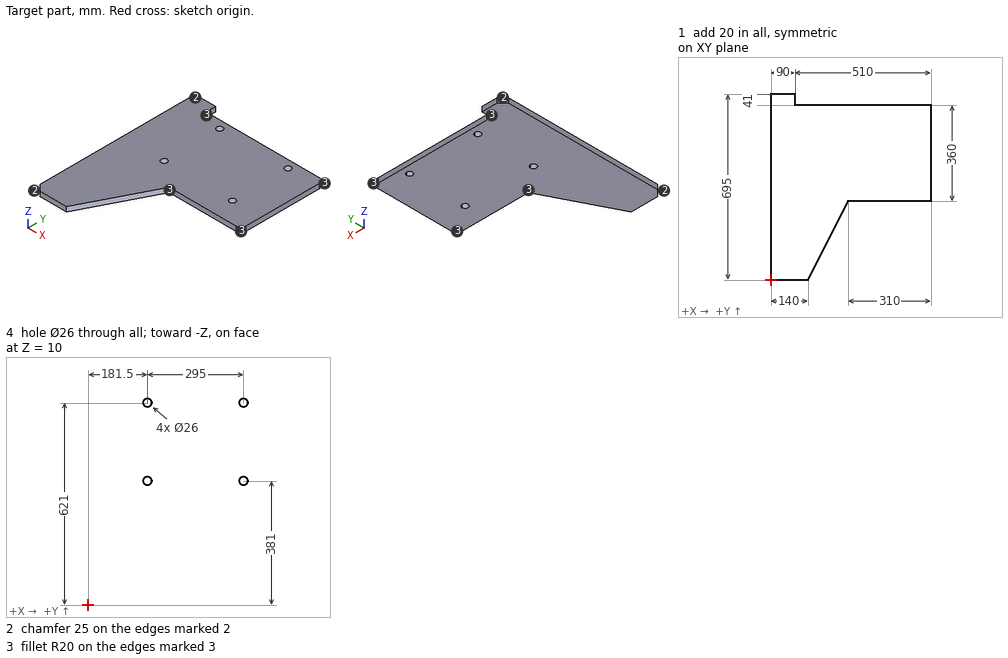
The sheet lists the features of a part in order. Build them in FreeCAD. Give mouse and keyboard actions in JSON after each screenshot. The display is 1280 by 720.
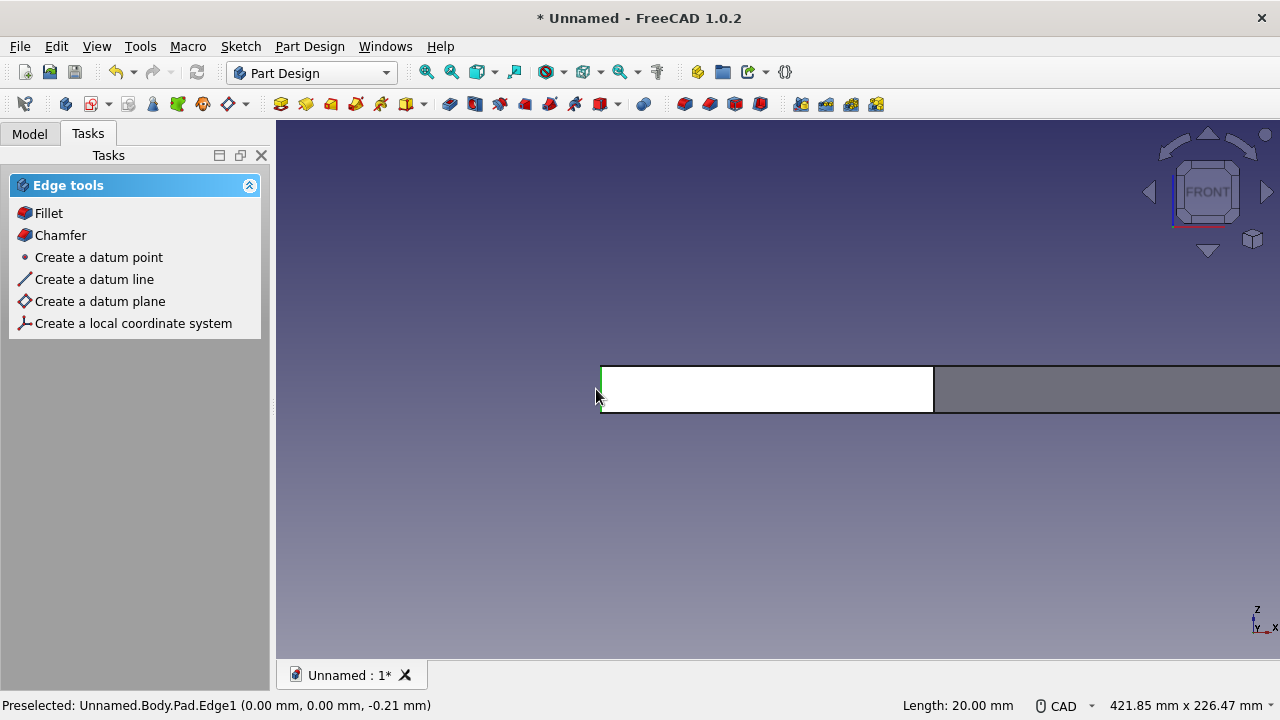
{"action": "left_click", "coordinate": [427, 72]}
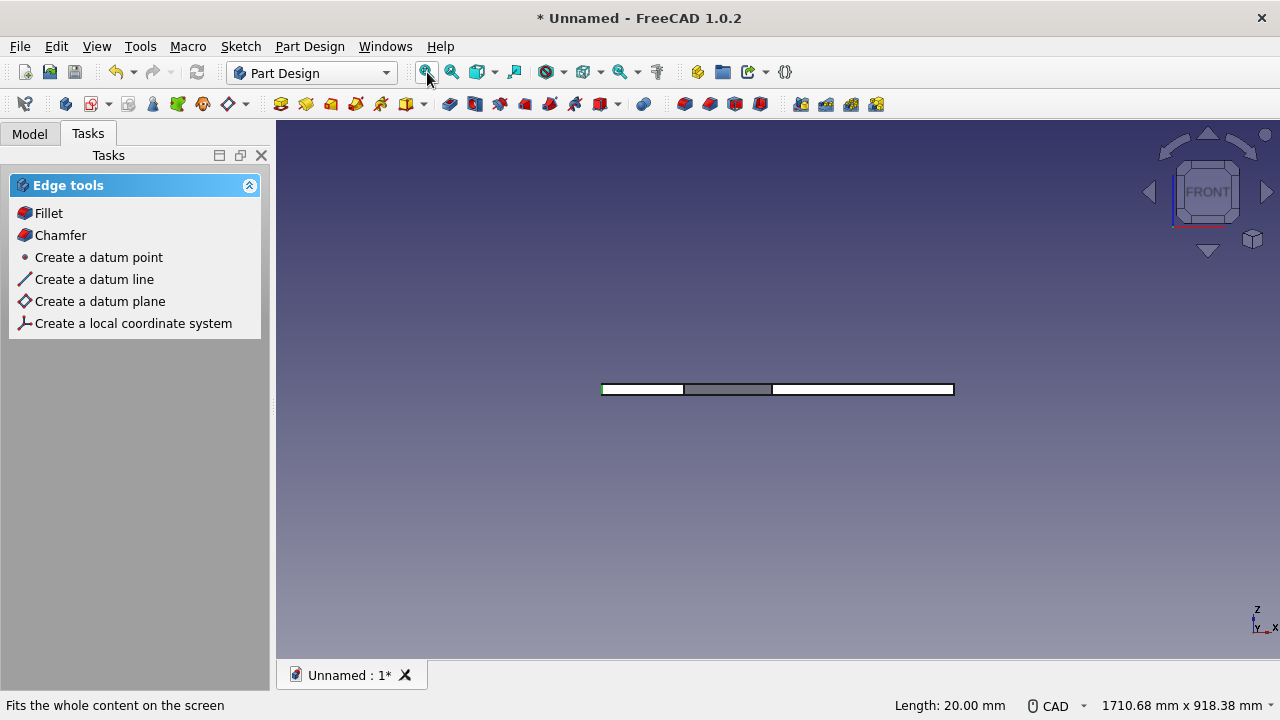
{"action": "key", "text": "3"}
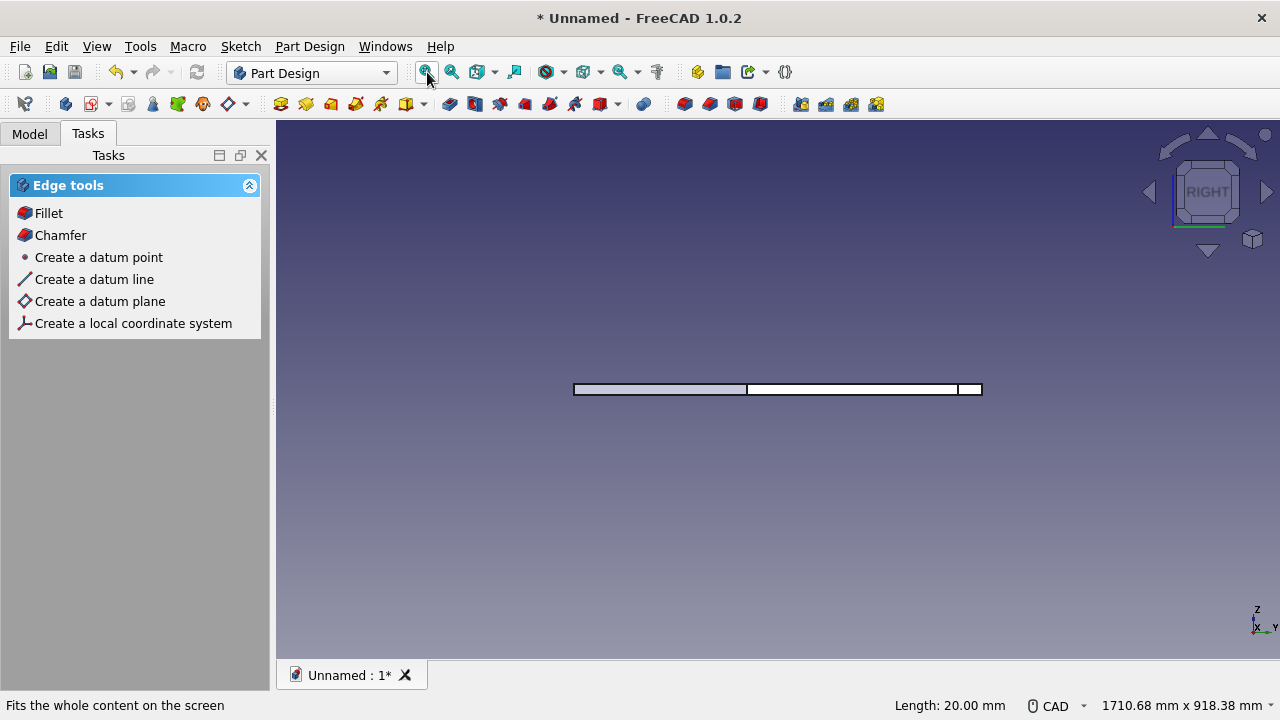
{"action": "left_click", "coordinate": [427, 72]}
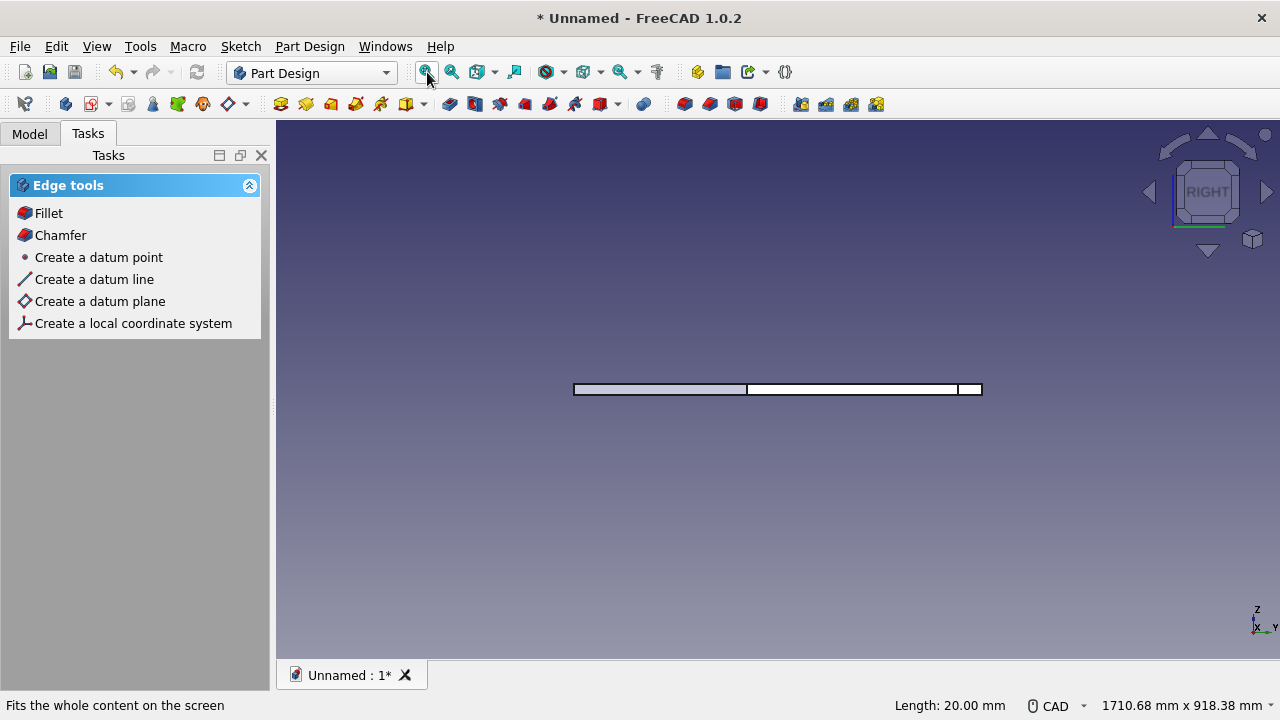
{"action": "scroll", "coordinate": [982, 388], "scroll_direction": "up", "scroll_amount": 7}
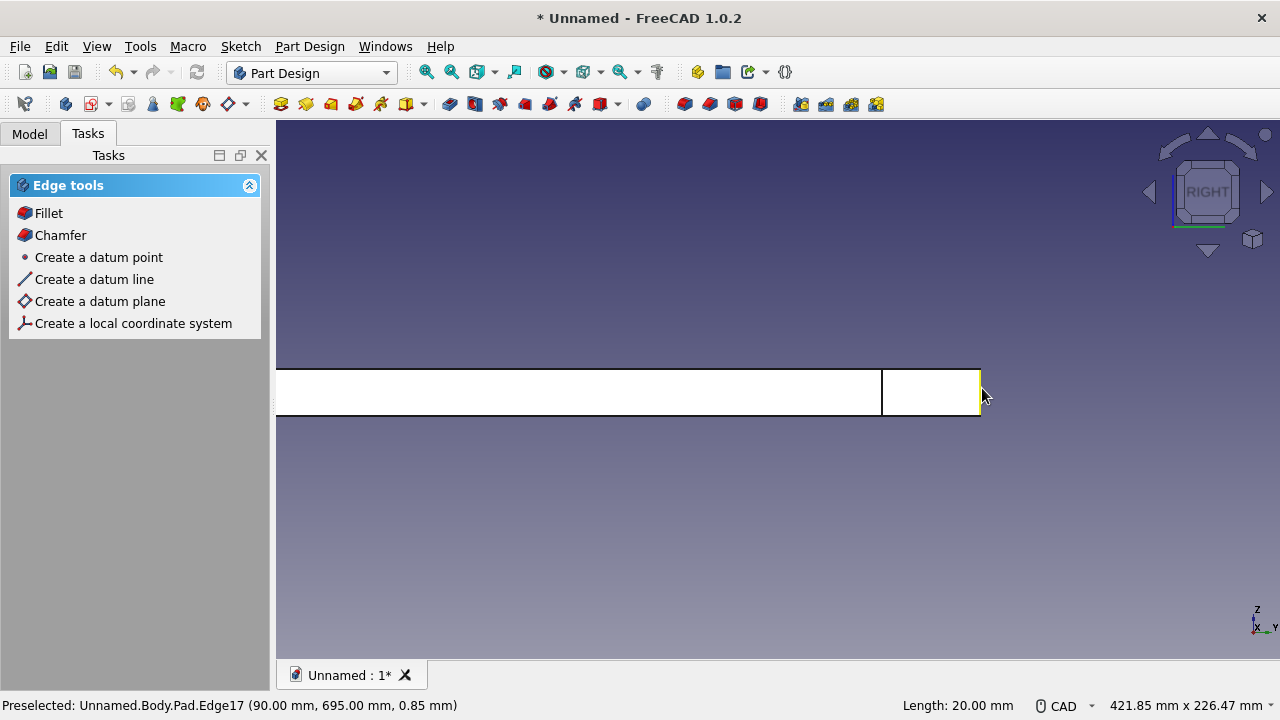
{"action": "left_click", "coordinate": [427, 72]}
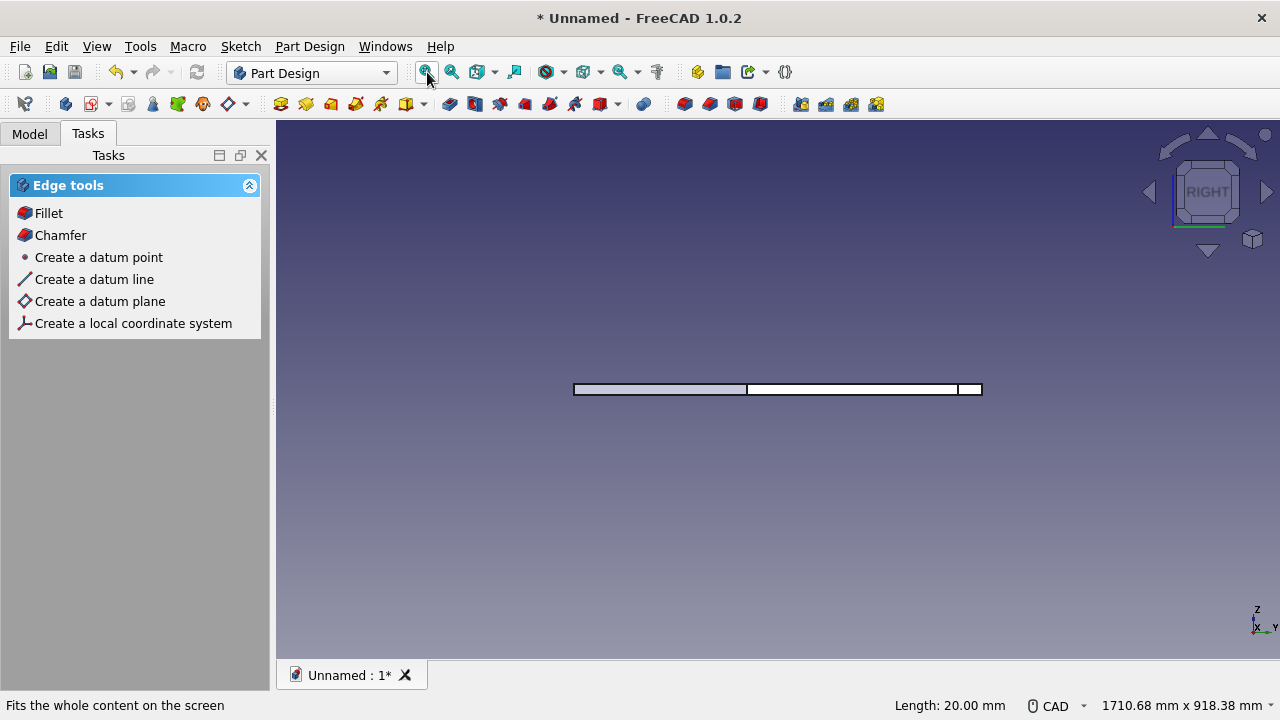
{"action": "key", "text": "5"}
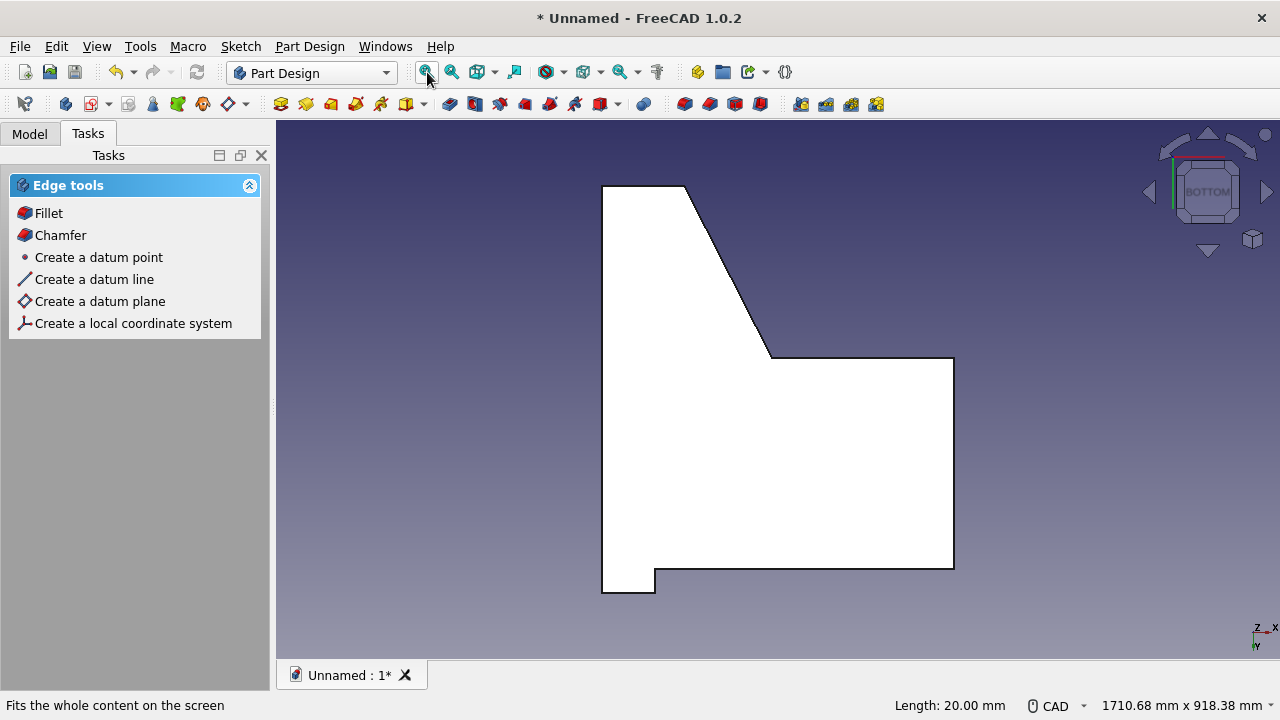
{"action": "scroll", "coordinate": [602, 592], "scroll_direction": "up", "scroll_amount": 7}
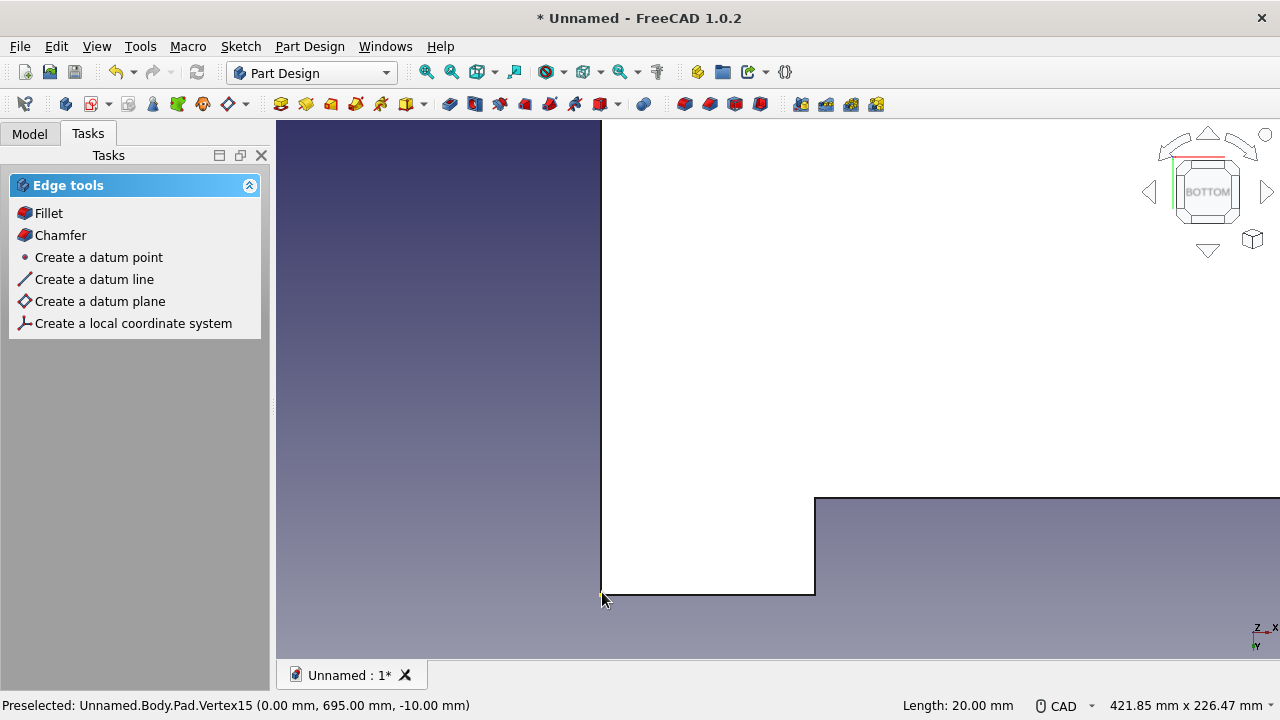
{"action": "left_click", "coordinate": [427, 72]}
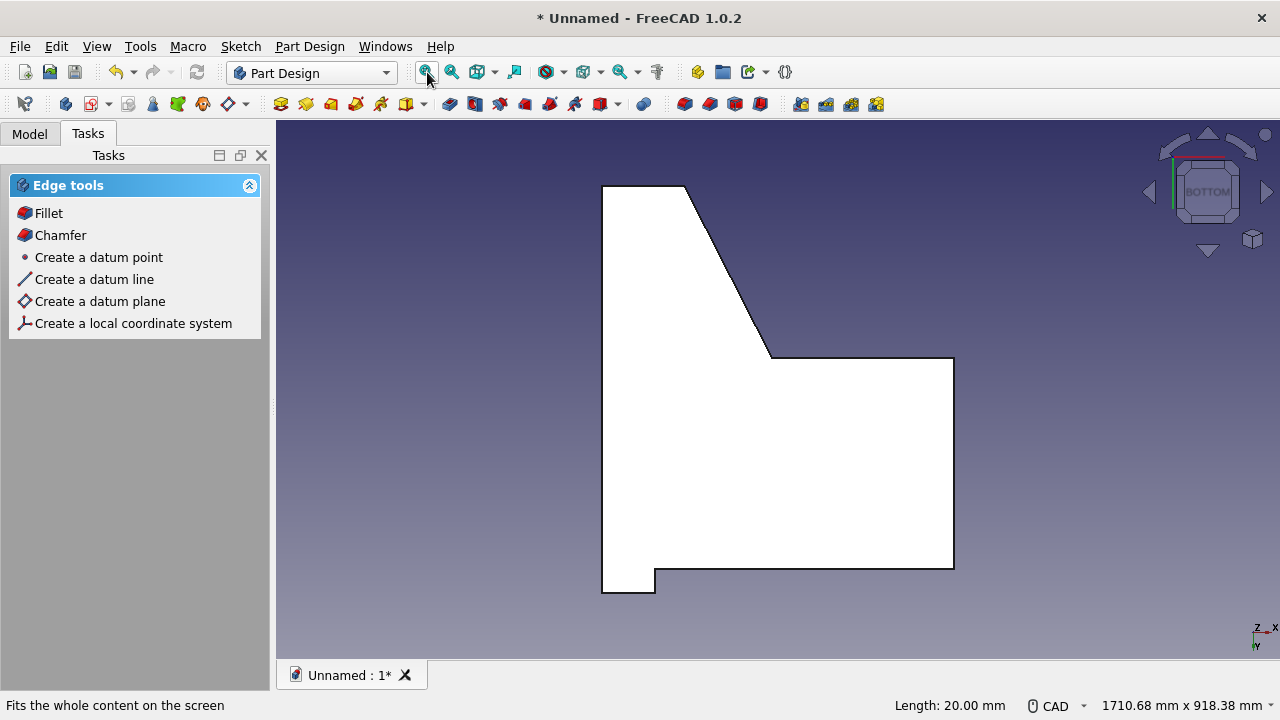
{"action": "key", "text": "4"}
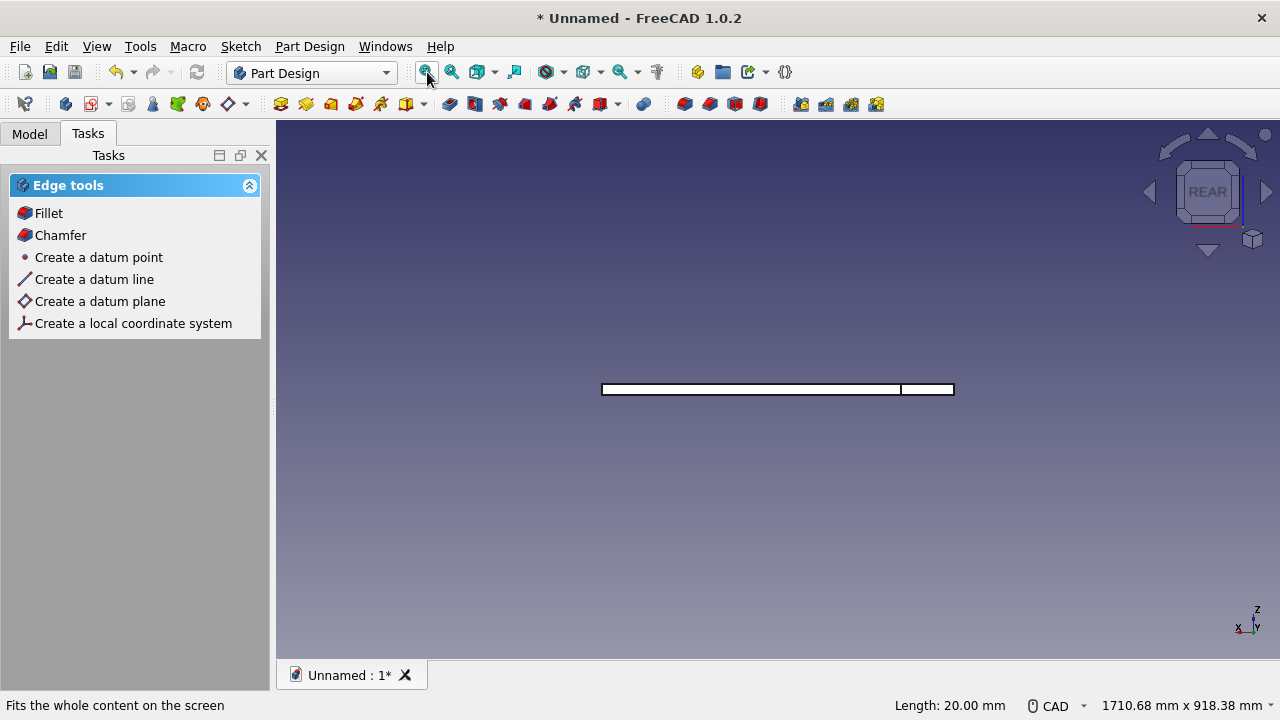
{"action": "left_click", "coordinate": [427, 72]}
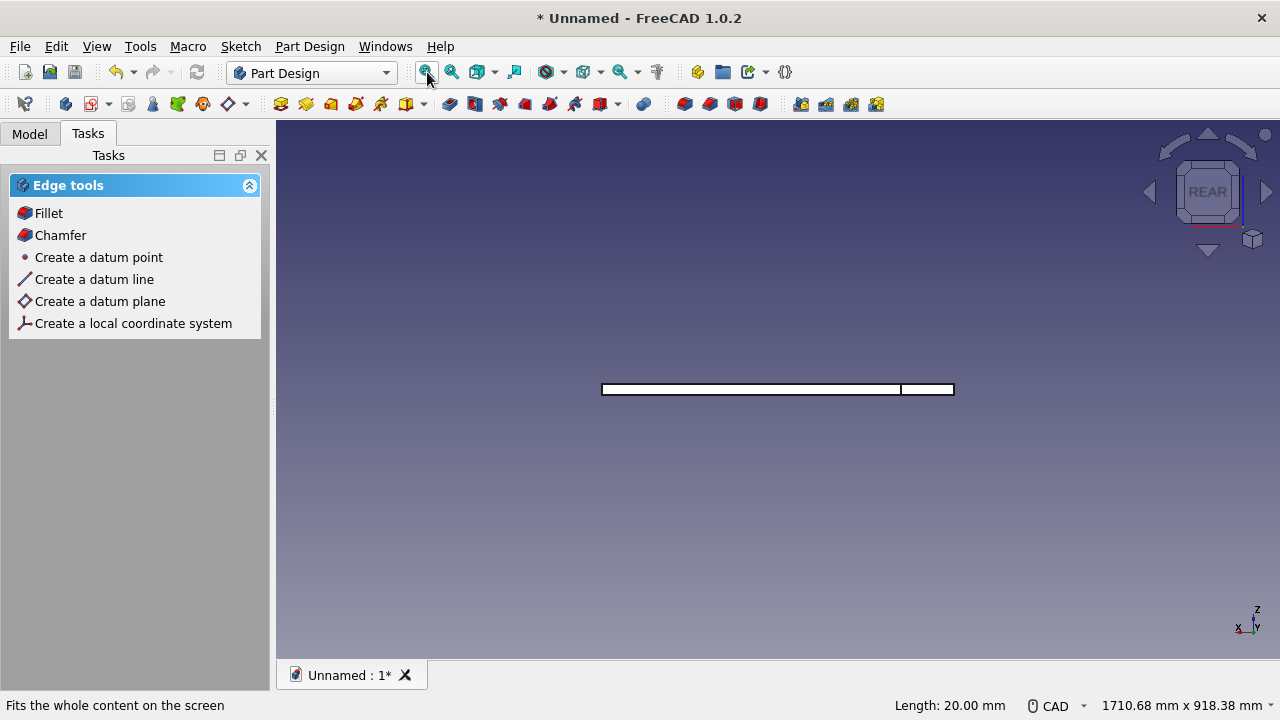
{"action": "scroll", "coordinate": [954, 389], "scroll_direction": "up", "scroll_amount": 7}